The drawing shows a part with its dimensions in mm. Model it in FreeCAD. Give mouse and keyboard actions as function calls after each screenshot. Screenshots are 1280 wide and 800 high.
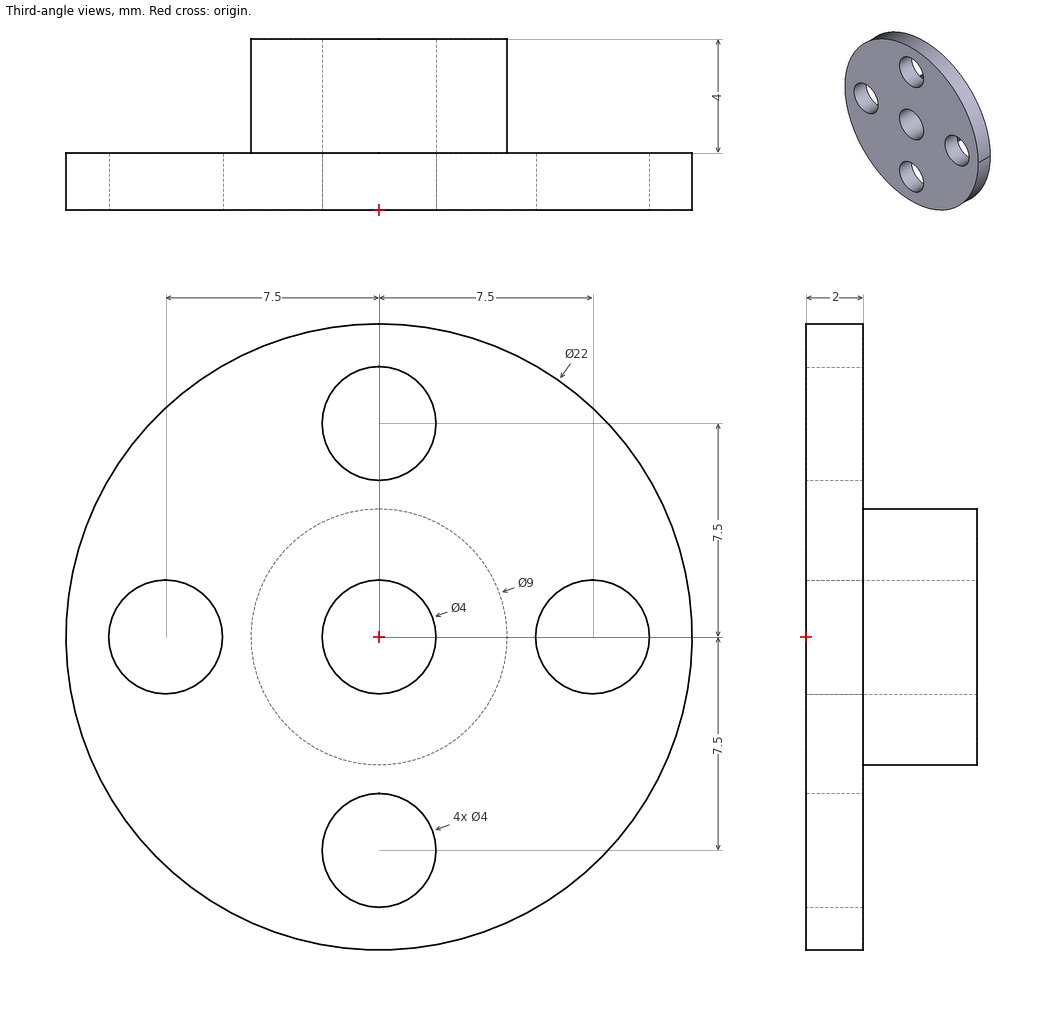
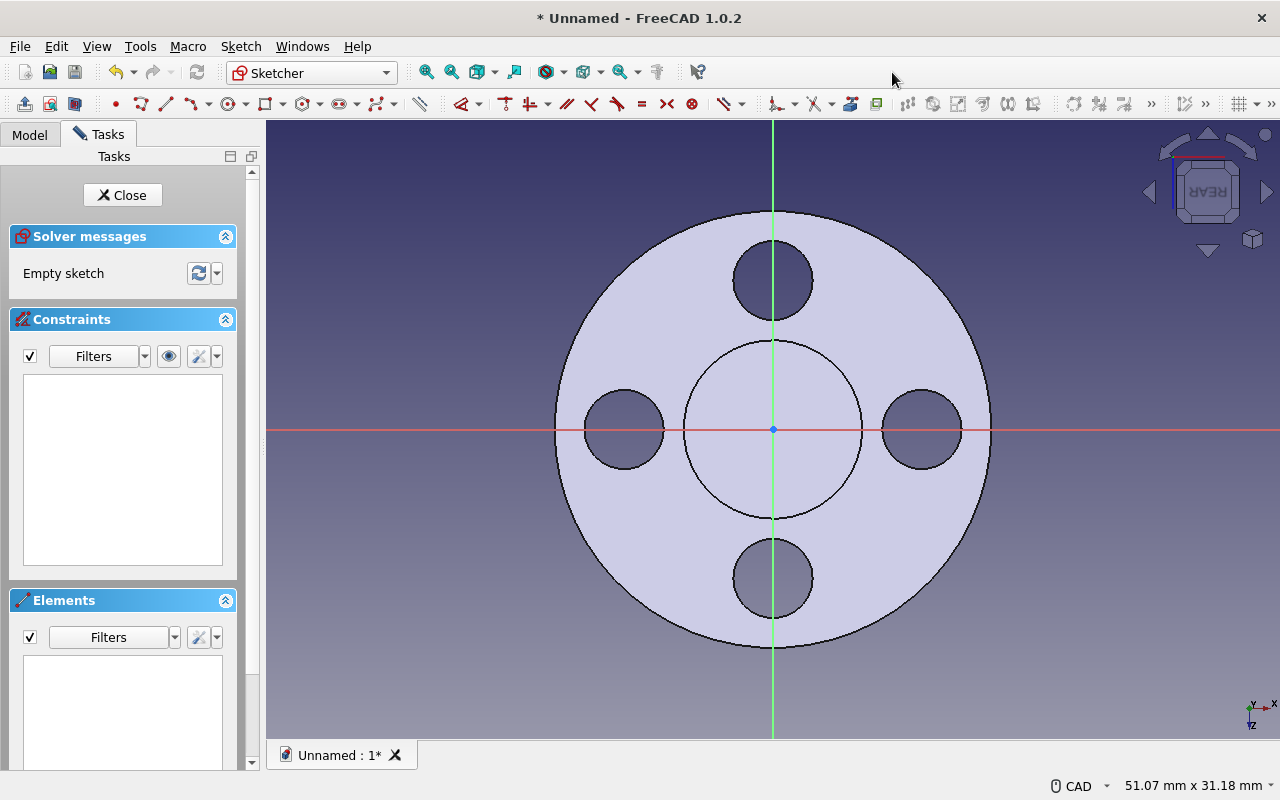
scroll(790, 429, up, 8)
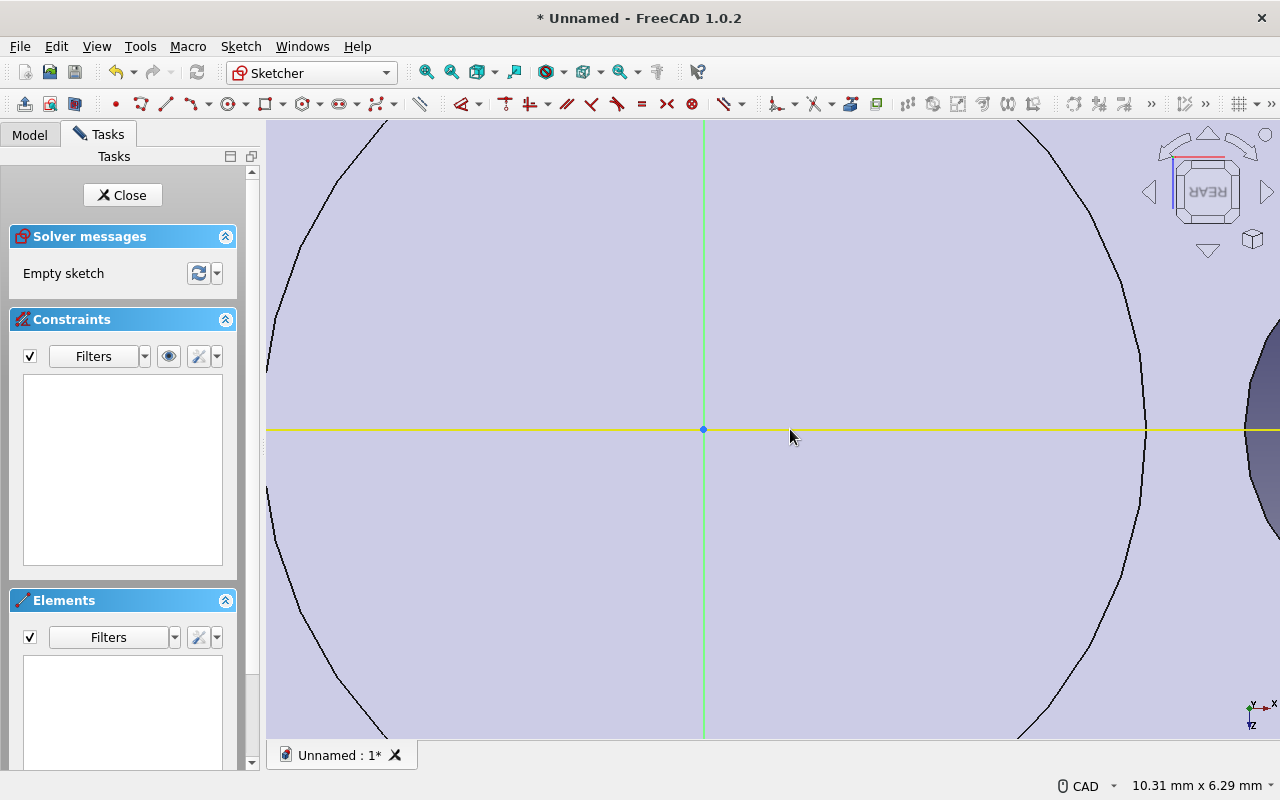
click(228, 104)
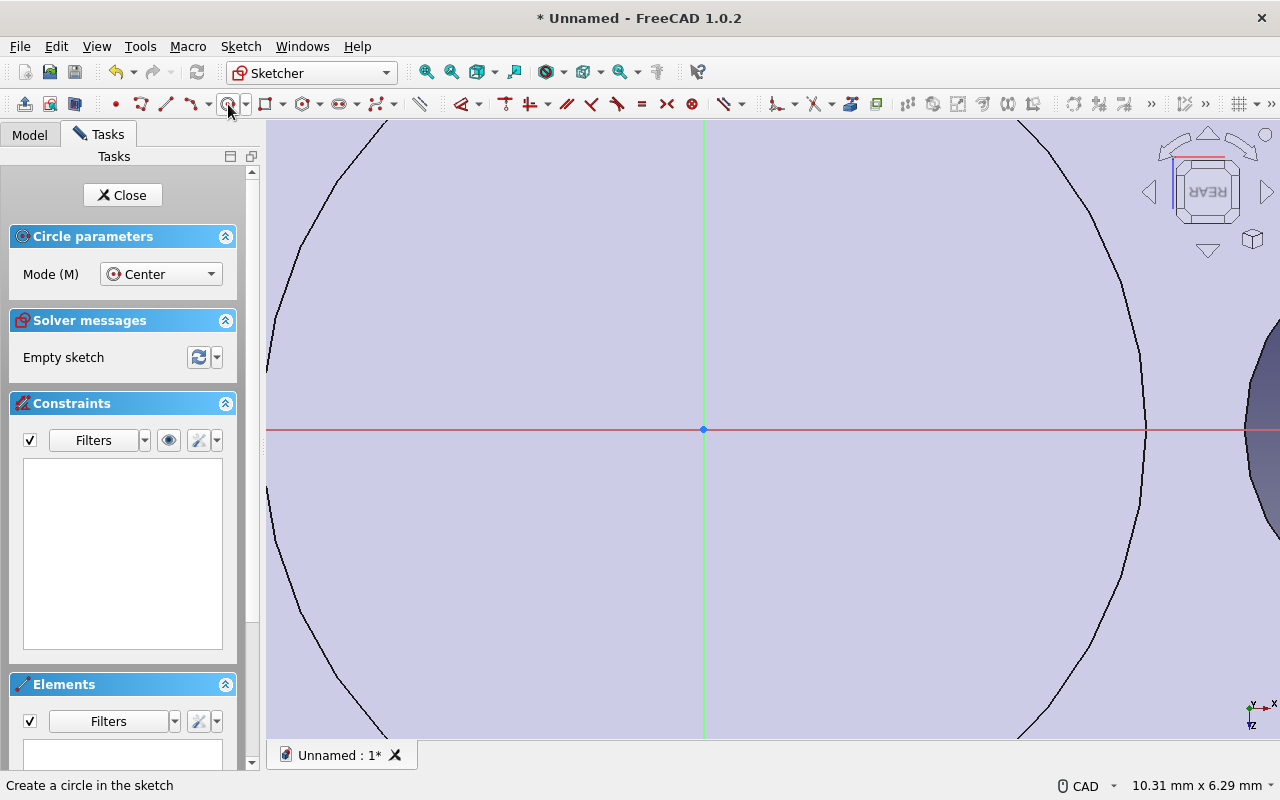
click(704, 429)
click(843, 290)
key(Escape)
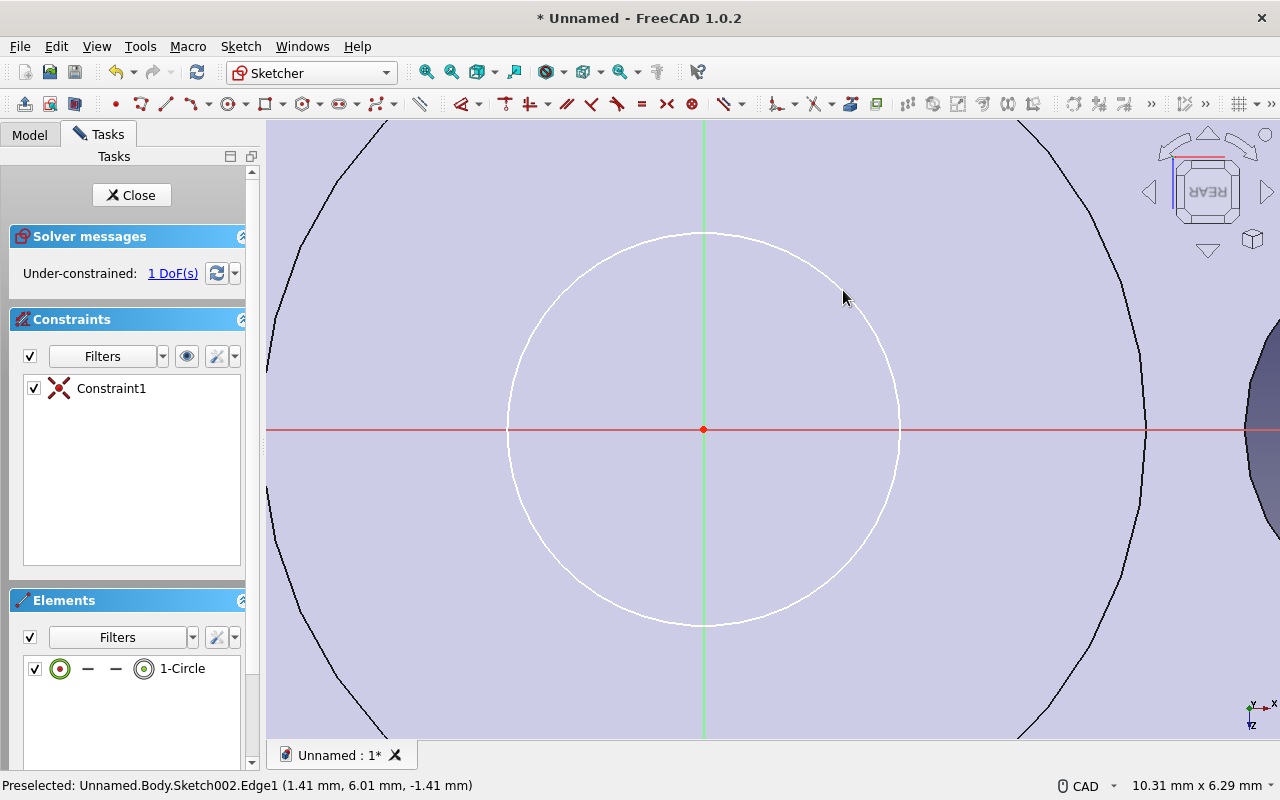
click(460, 104)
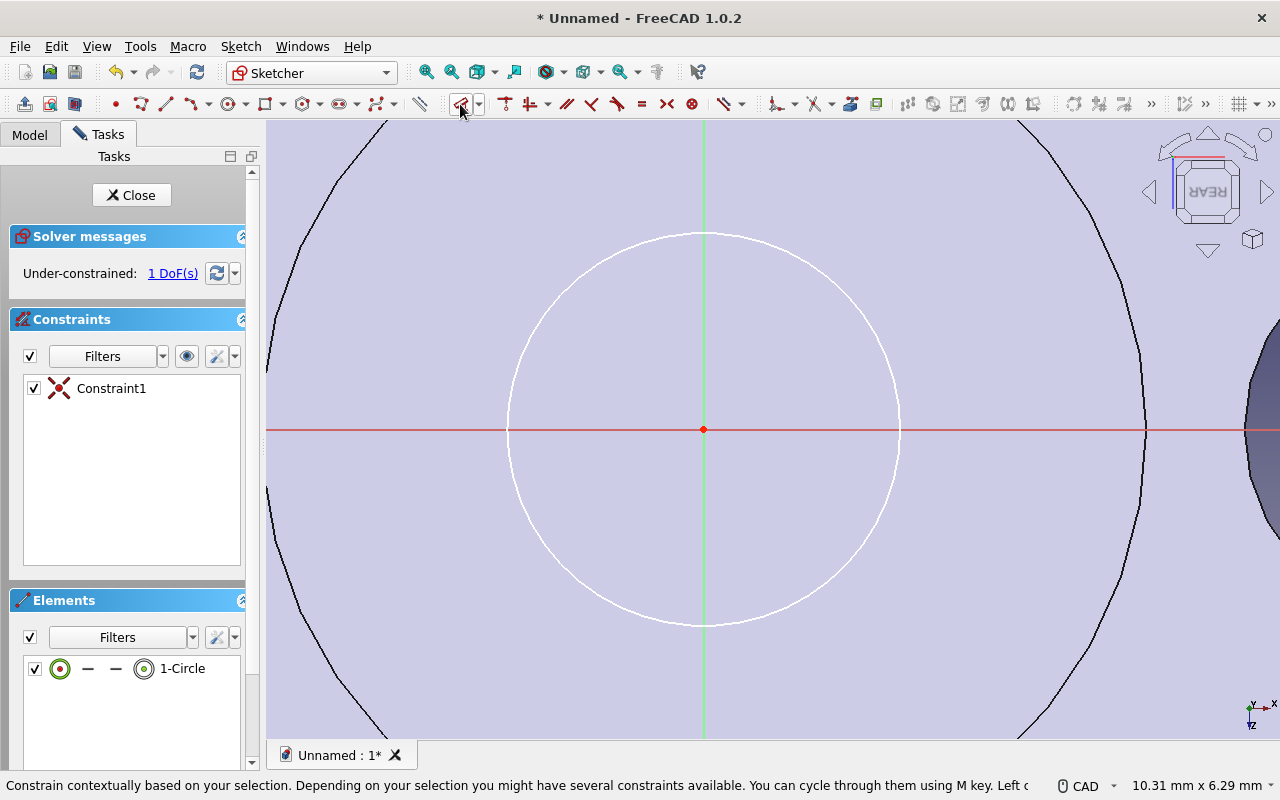
click(842, 290)
click(865, 267)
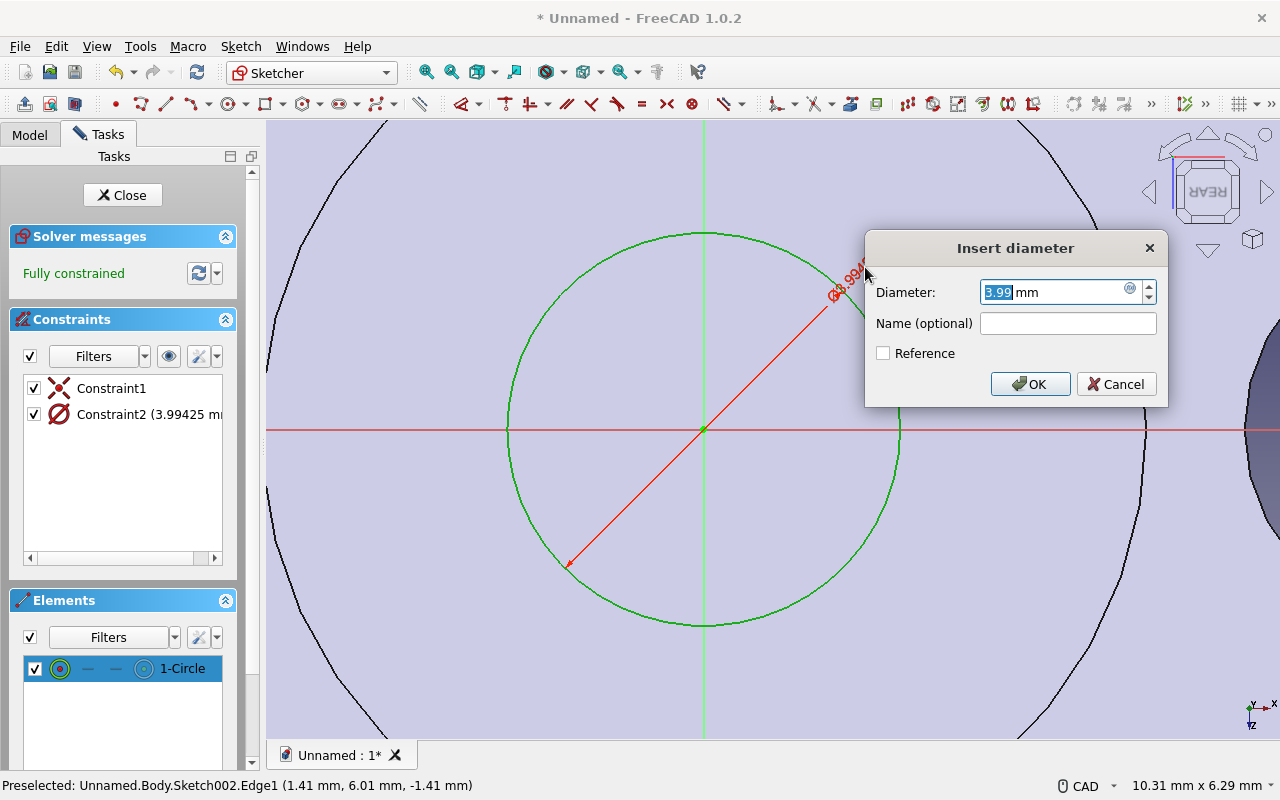
text(4)
key(Return)
key(Escape)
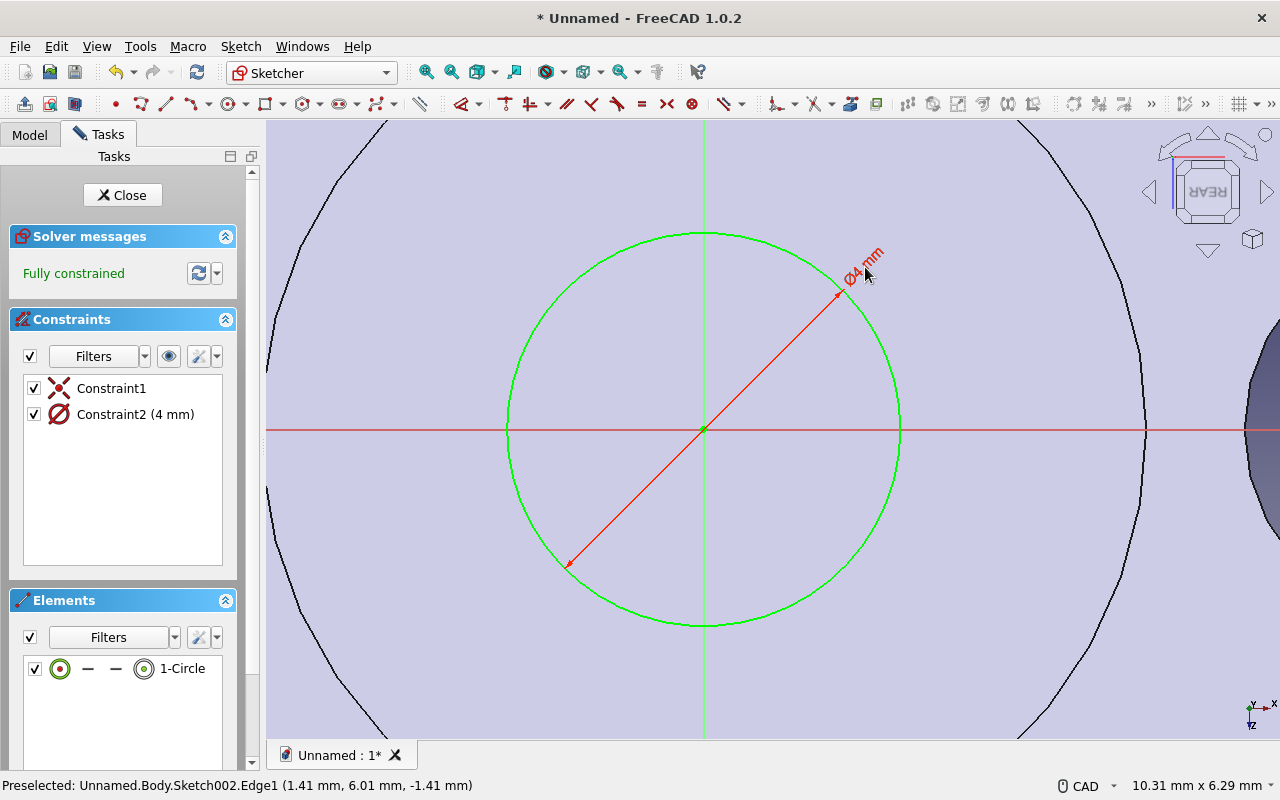
click(123, 195)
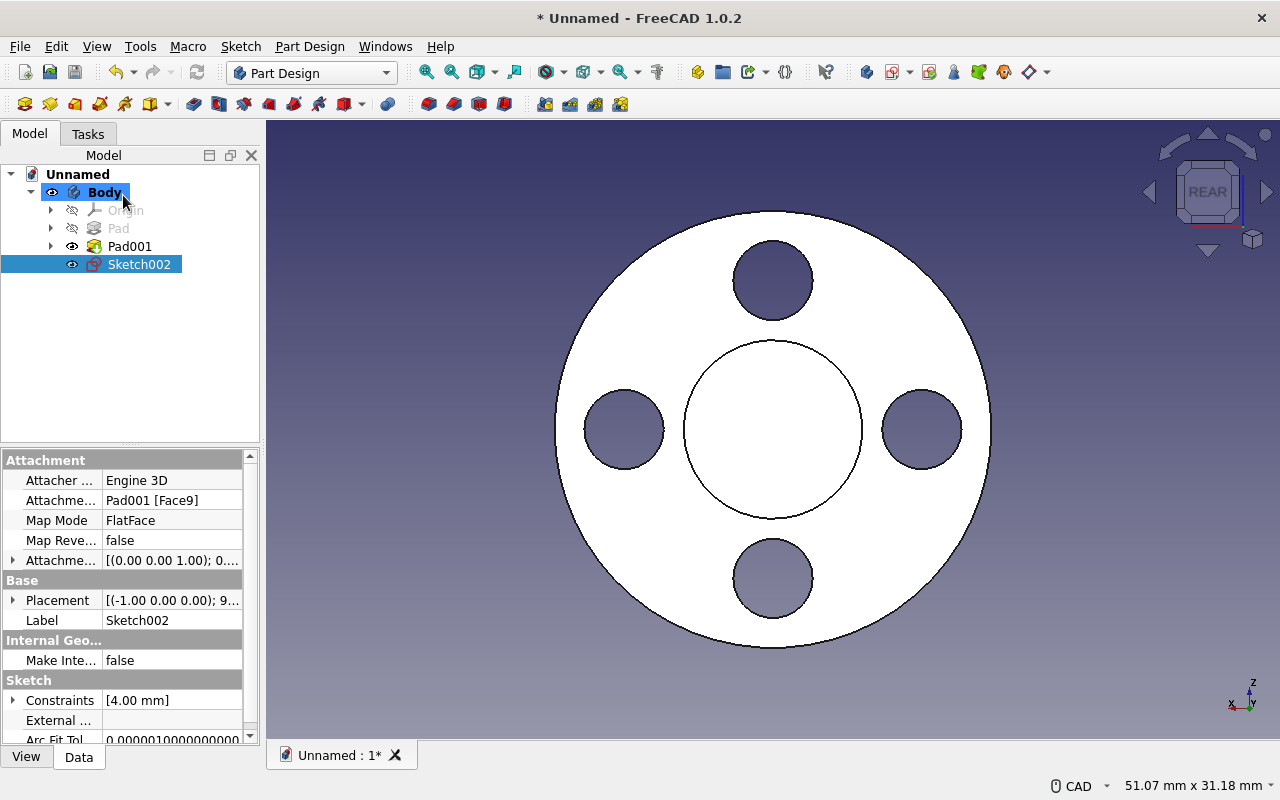
click(194, 104)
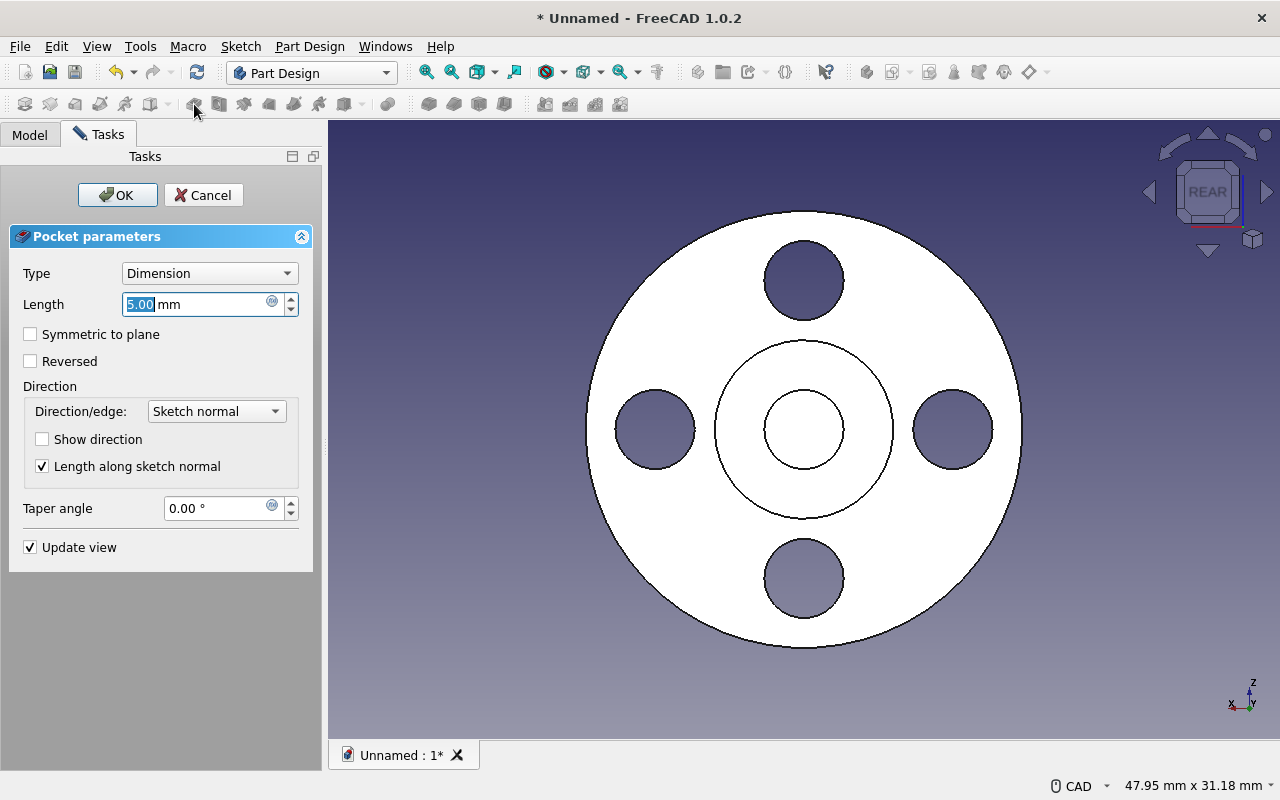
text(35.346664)
key(Tab)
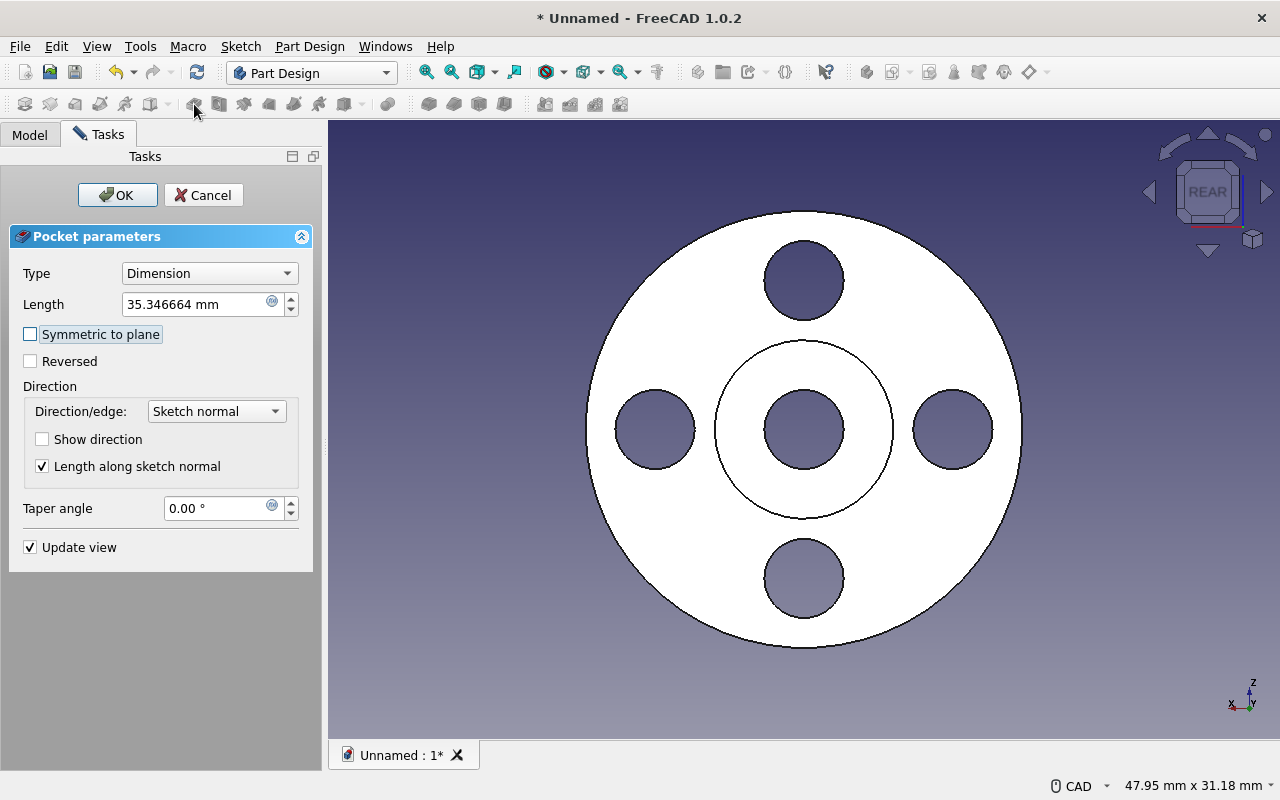
click(31, 334)